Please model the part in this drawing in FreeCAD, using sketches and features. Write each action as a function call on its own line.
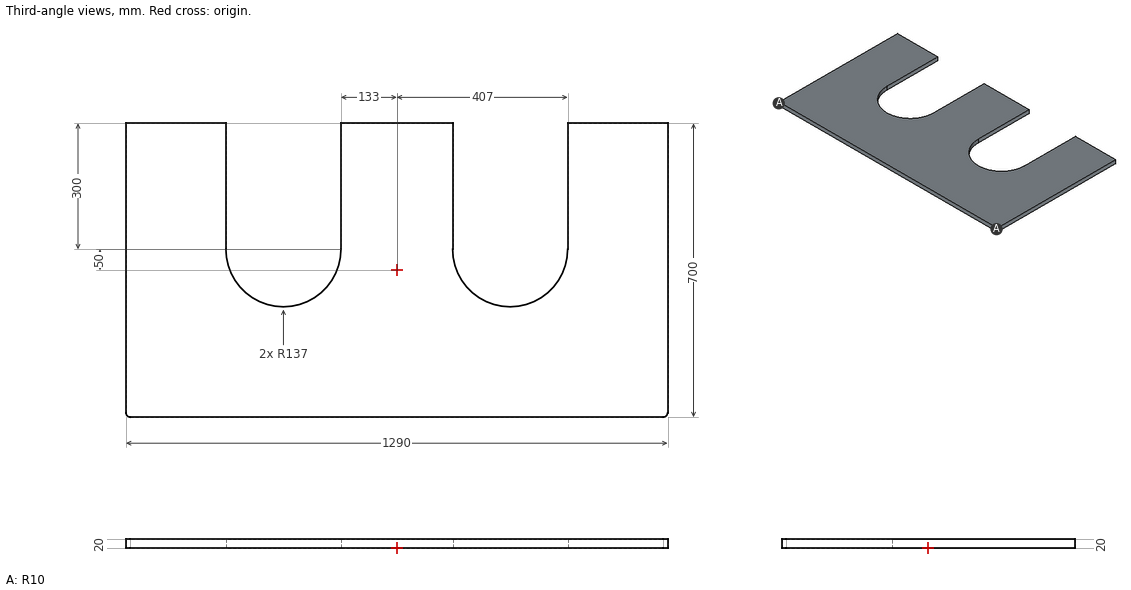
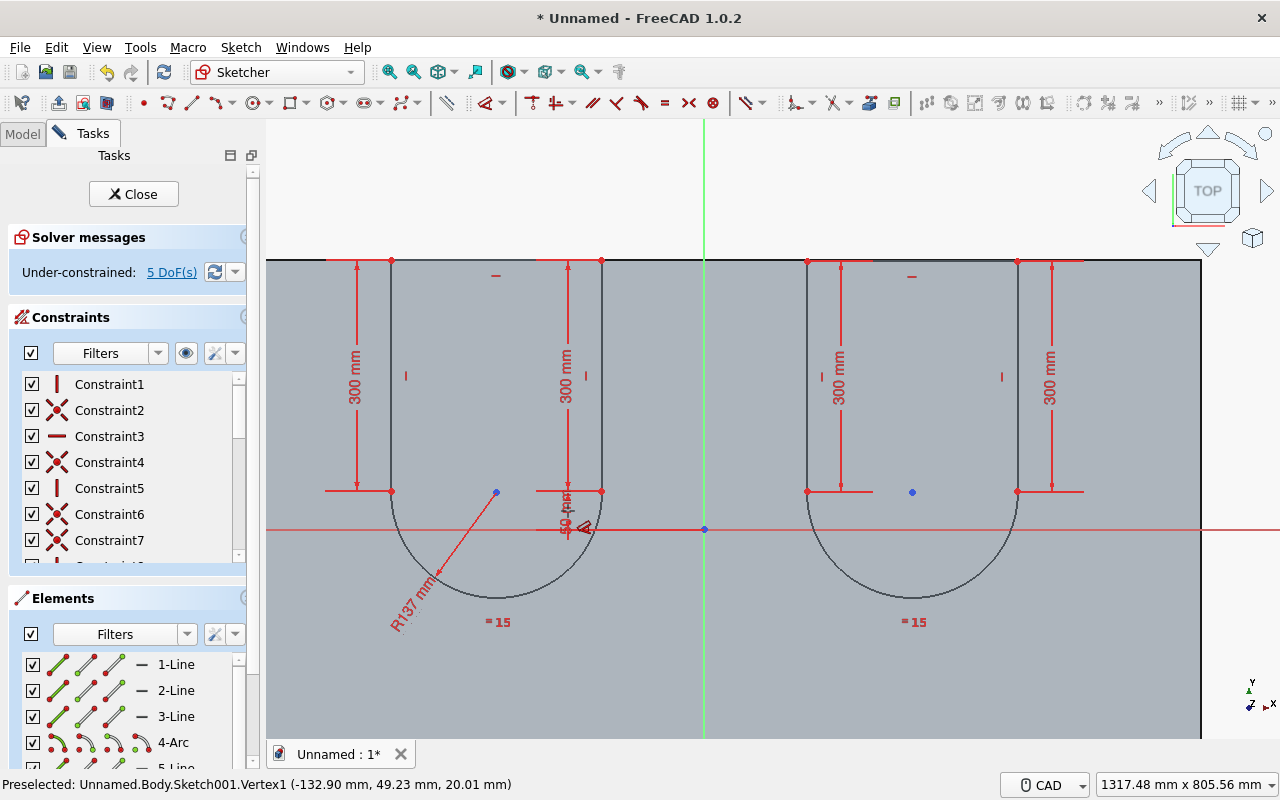
click(1018, 492)
click(1052, 511)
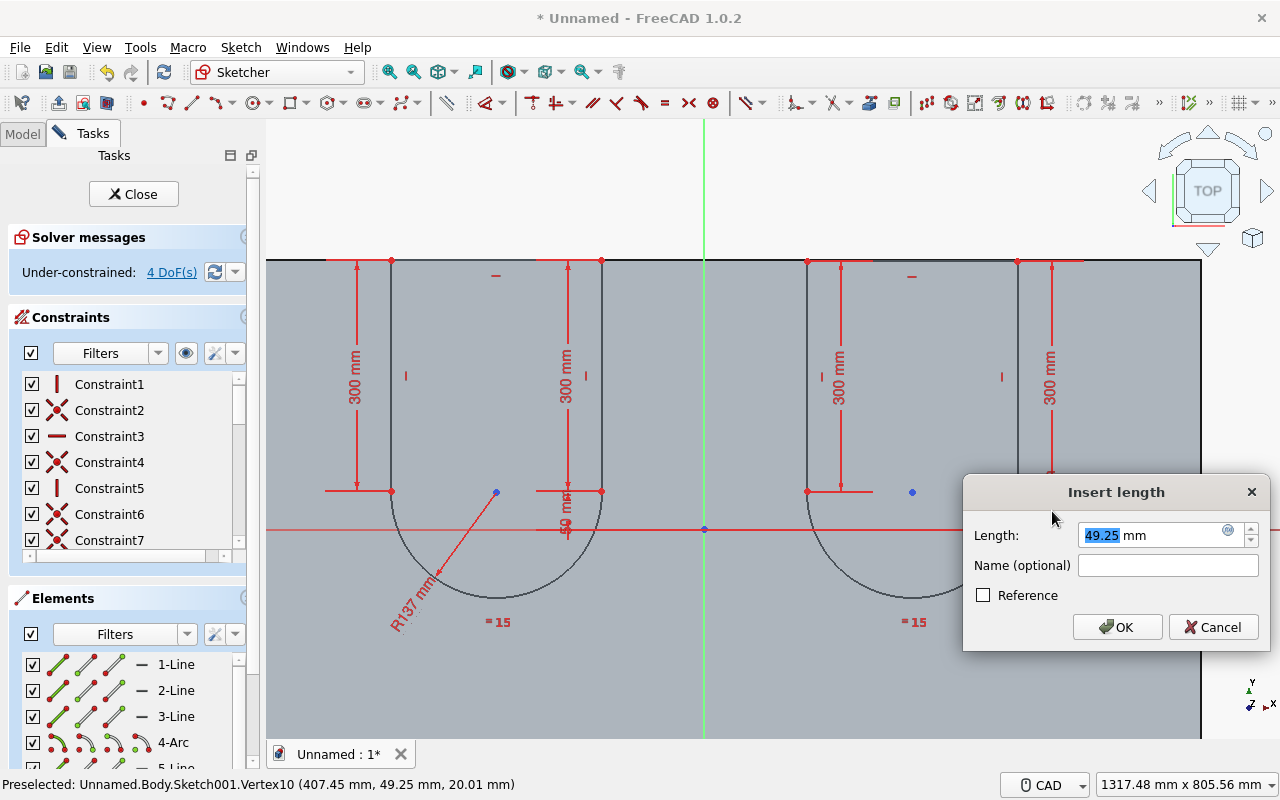
text(50)
key(Return)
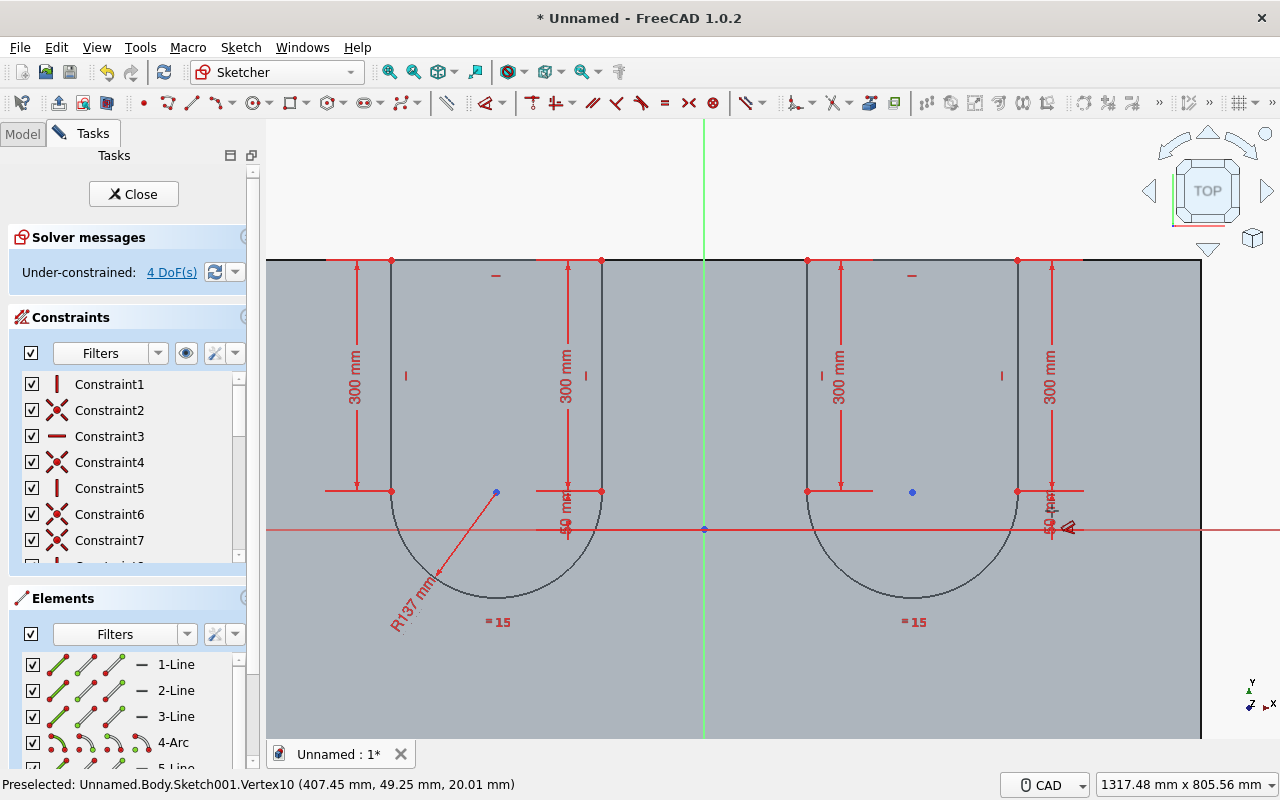
click(497, 492)
click(463, 511)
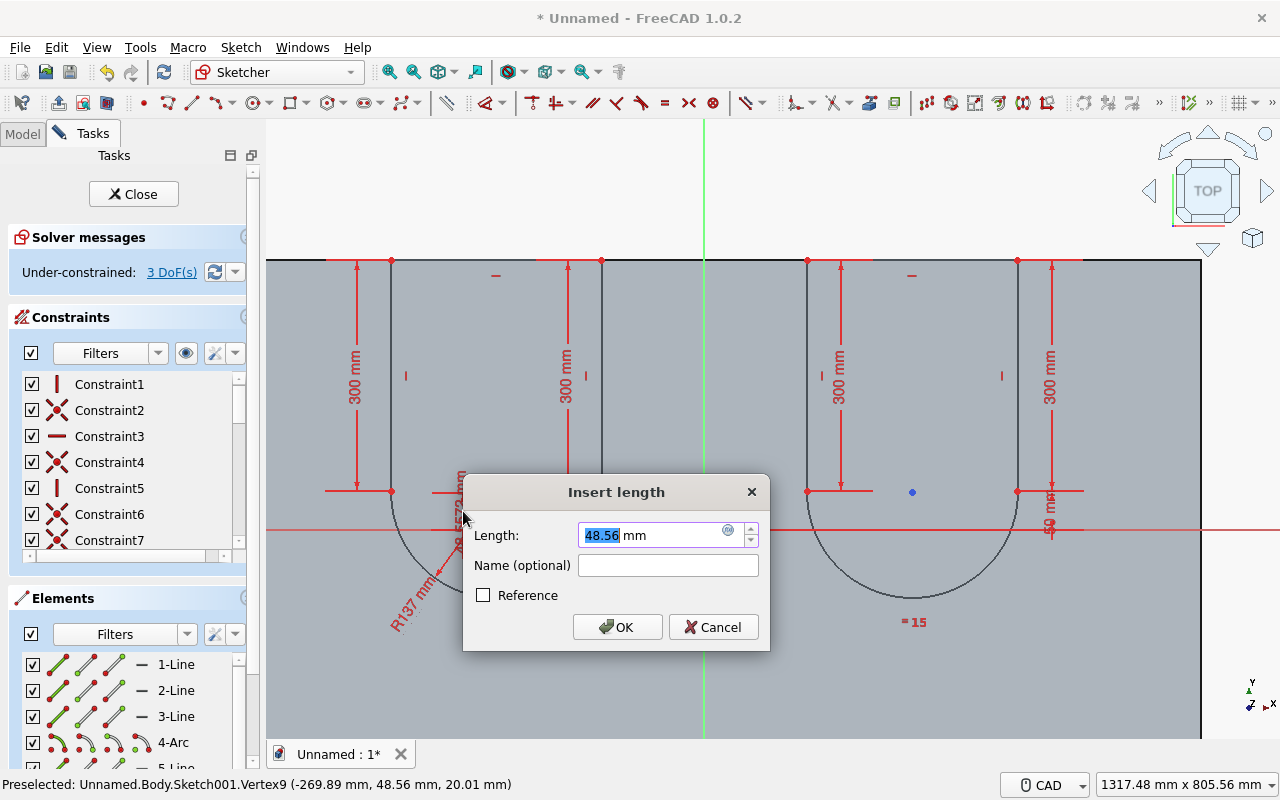
text(50)
key(Return)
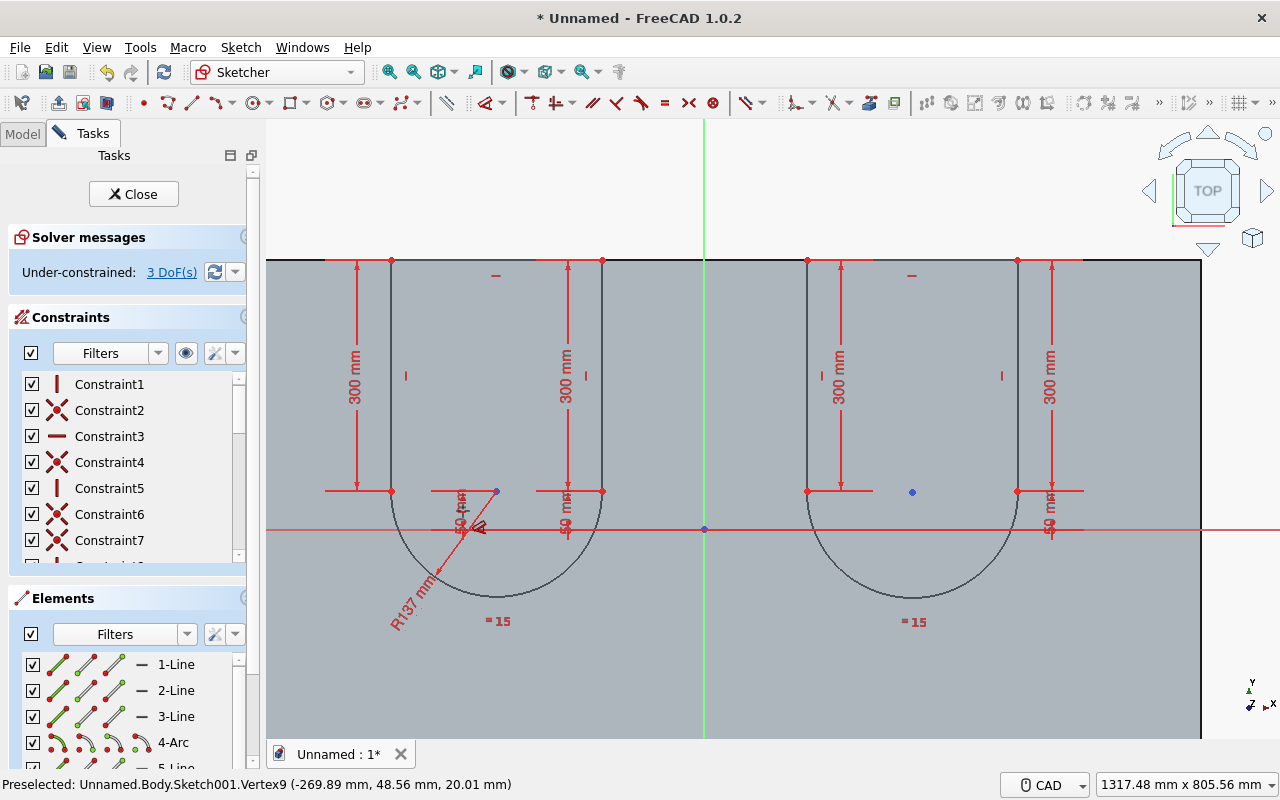
click(912, 492)
click(946, 511)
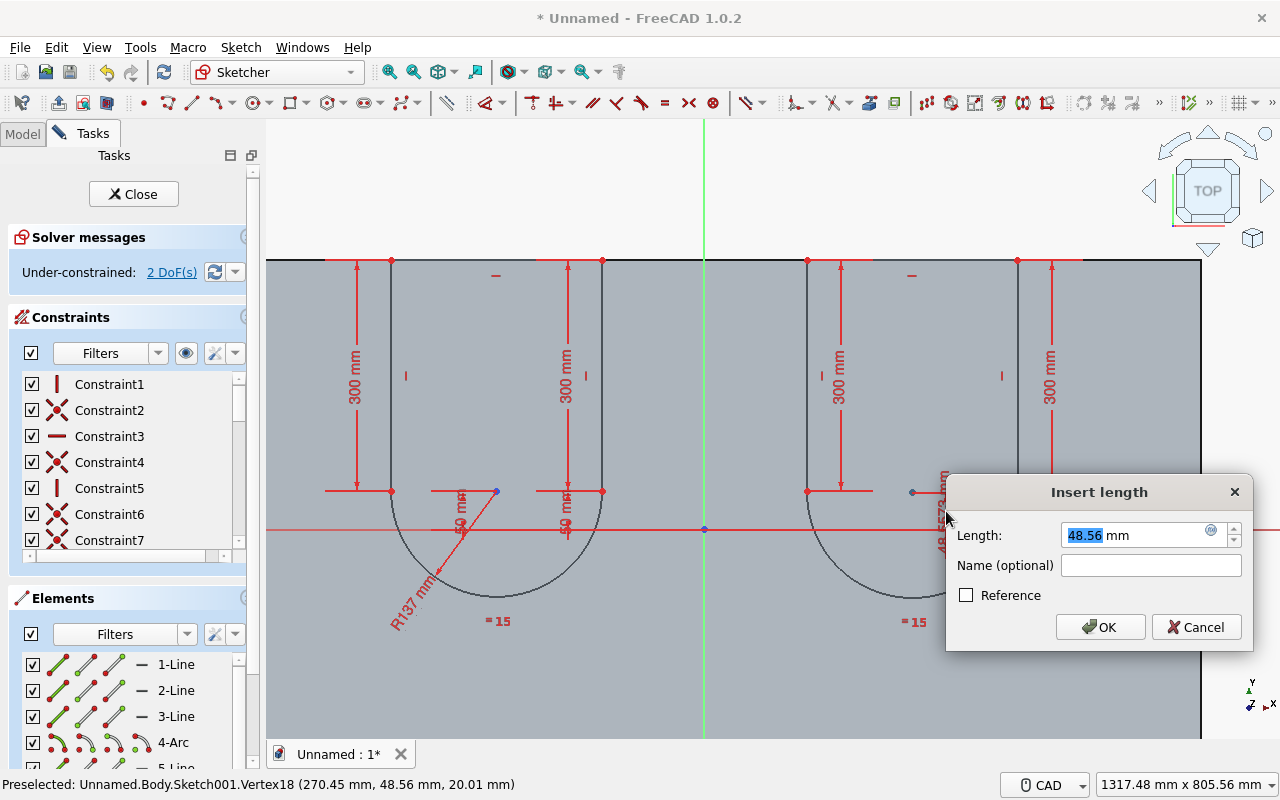
text(50)
key(Return)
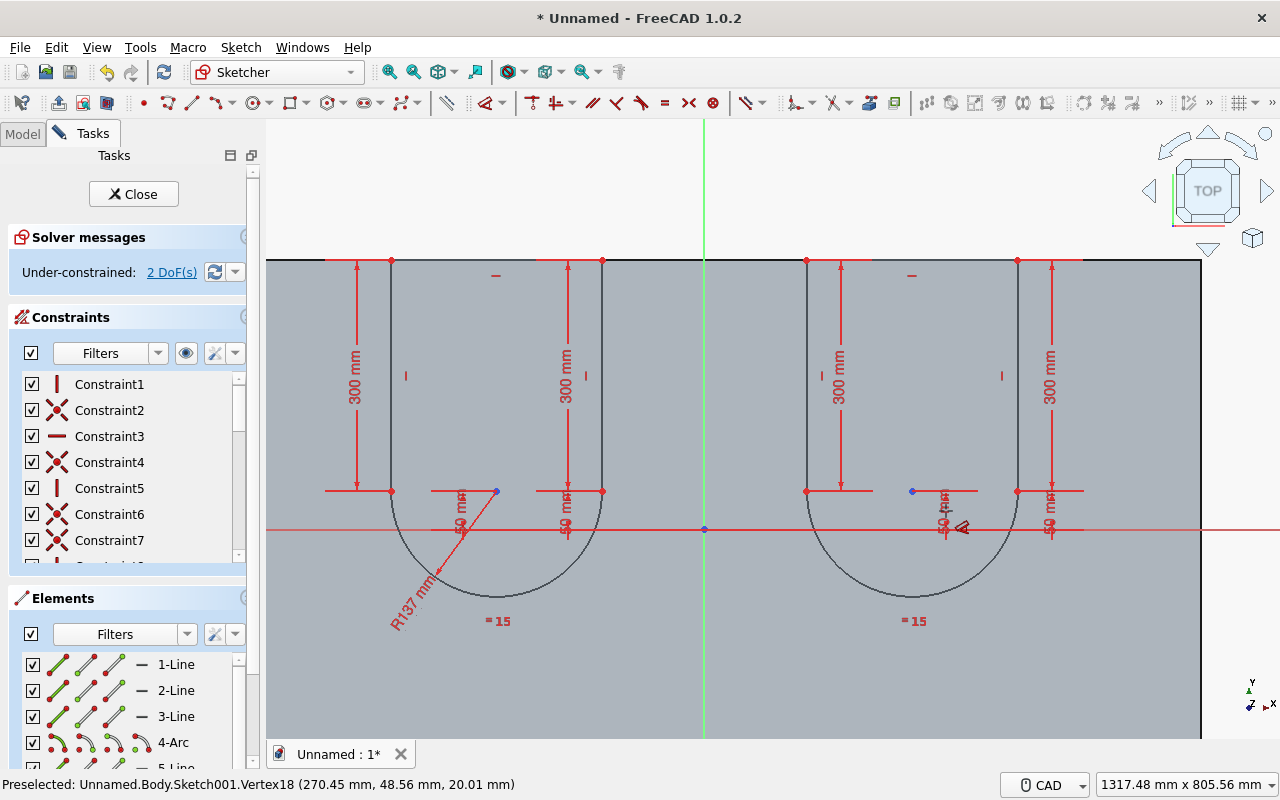
click(602, 491)
click(653, 564)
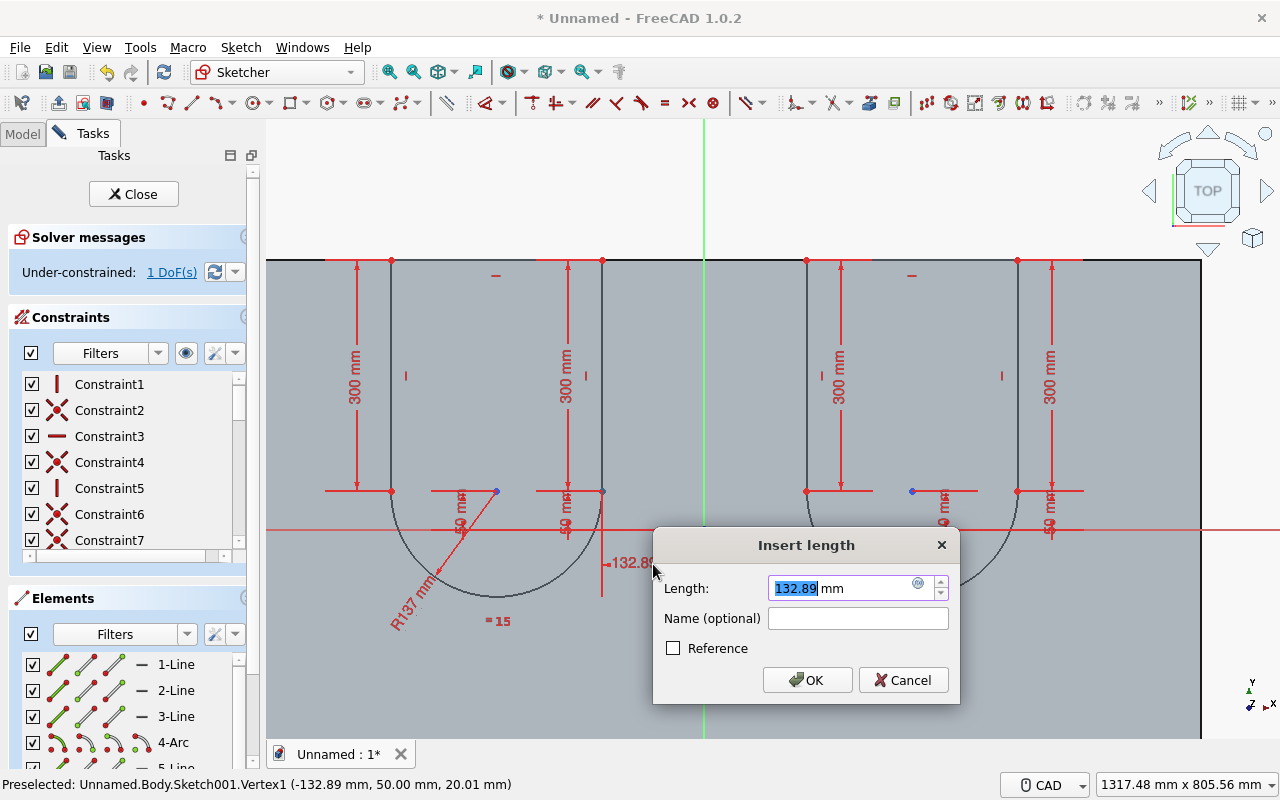
text(133)
key(Return)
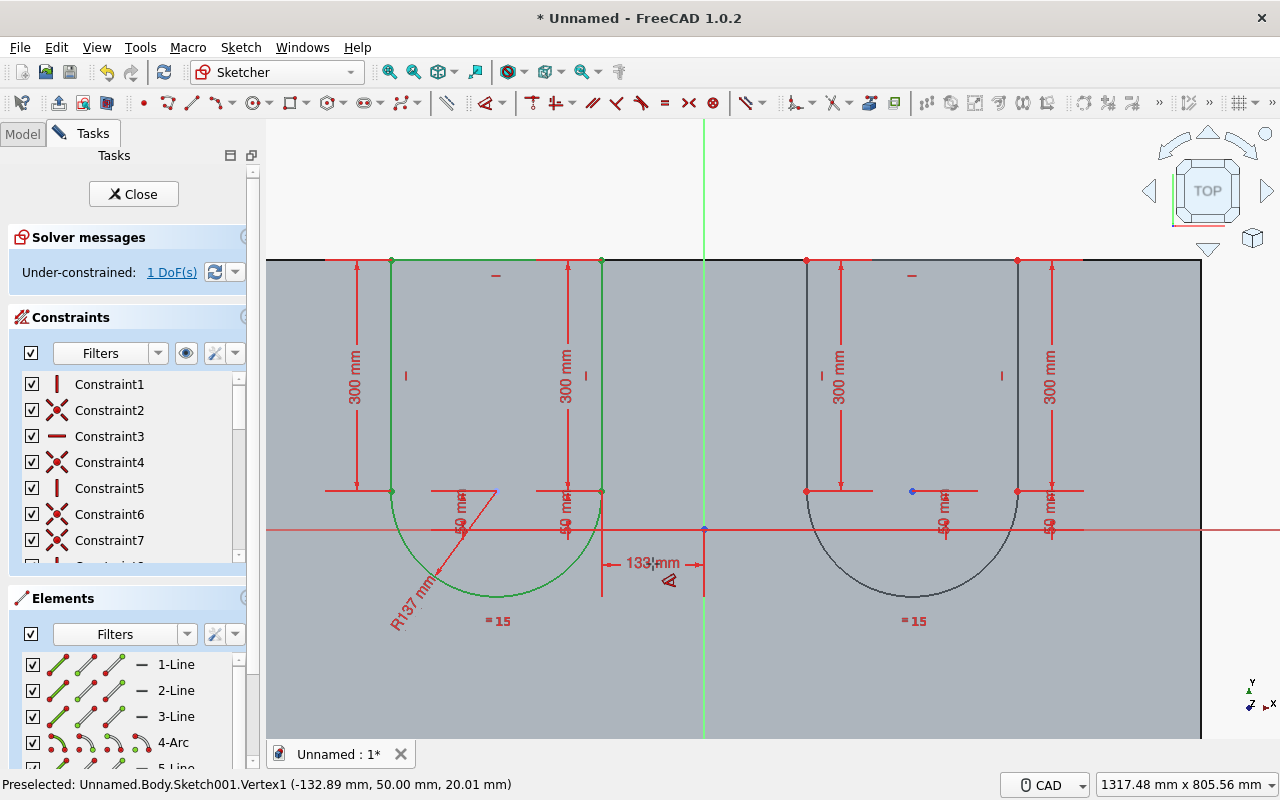
click(1018, 491)
click(861, 564)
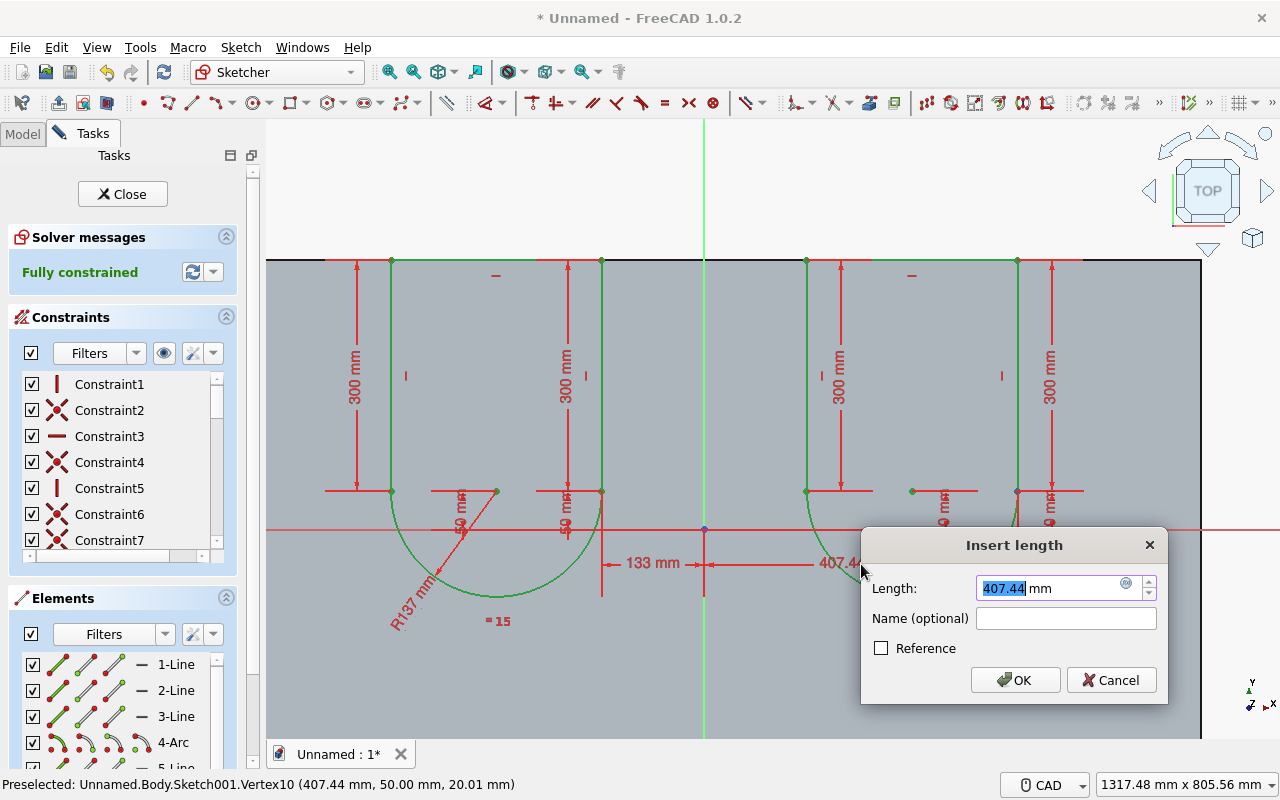
text(407)
key(Return)
key(Escape)